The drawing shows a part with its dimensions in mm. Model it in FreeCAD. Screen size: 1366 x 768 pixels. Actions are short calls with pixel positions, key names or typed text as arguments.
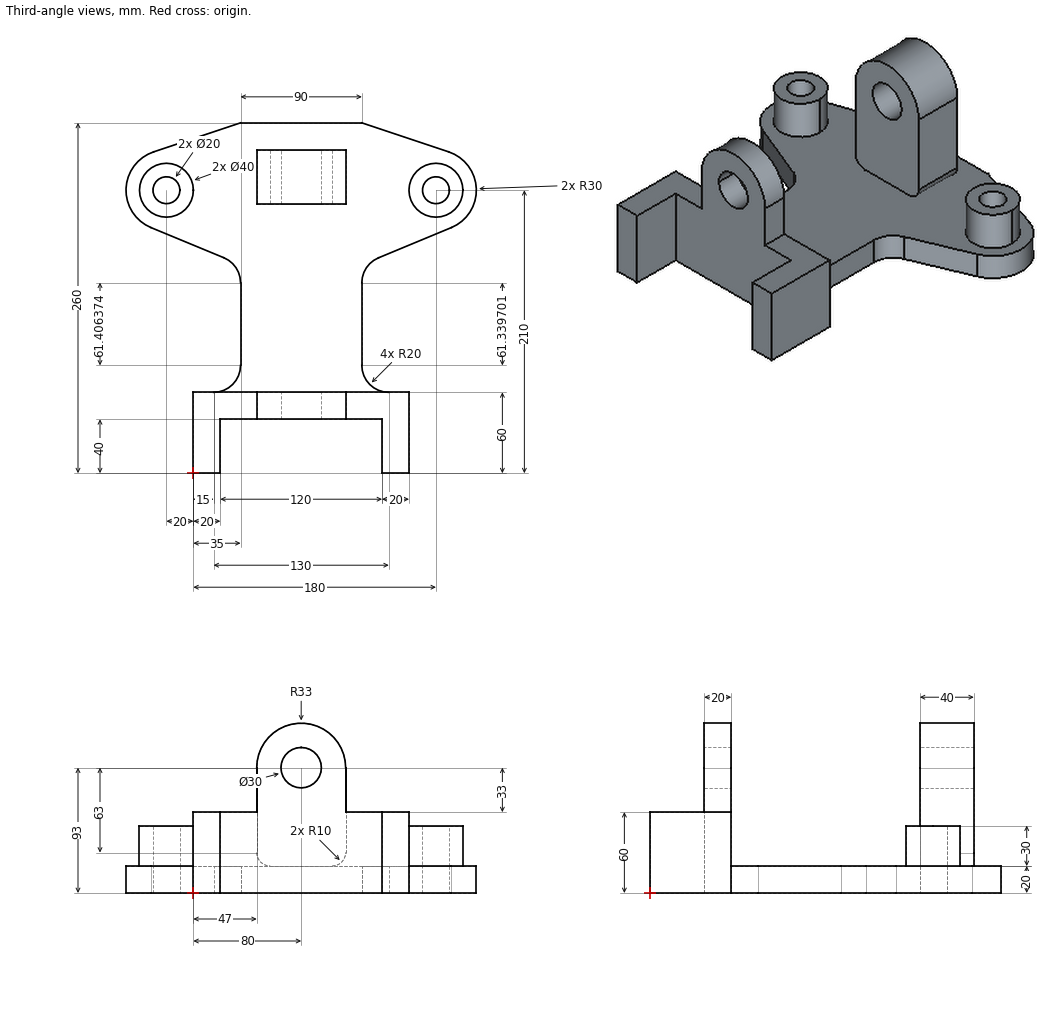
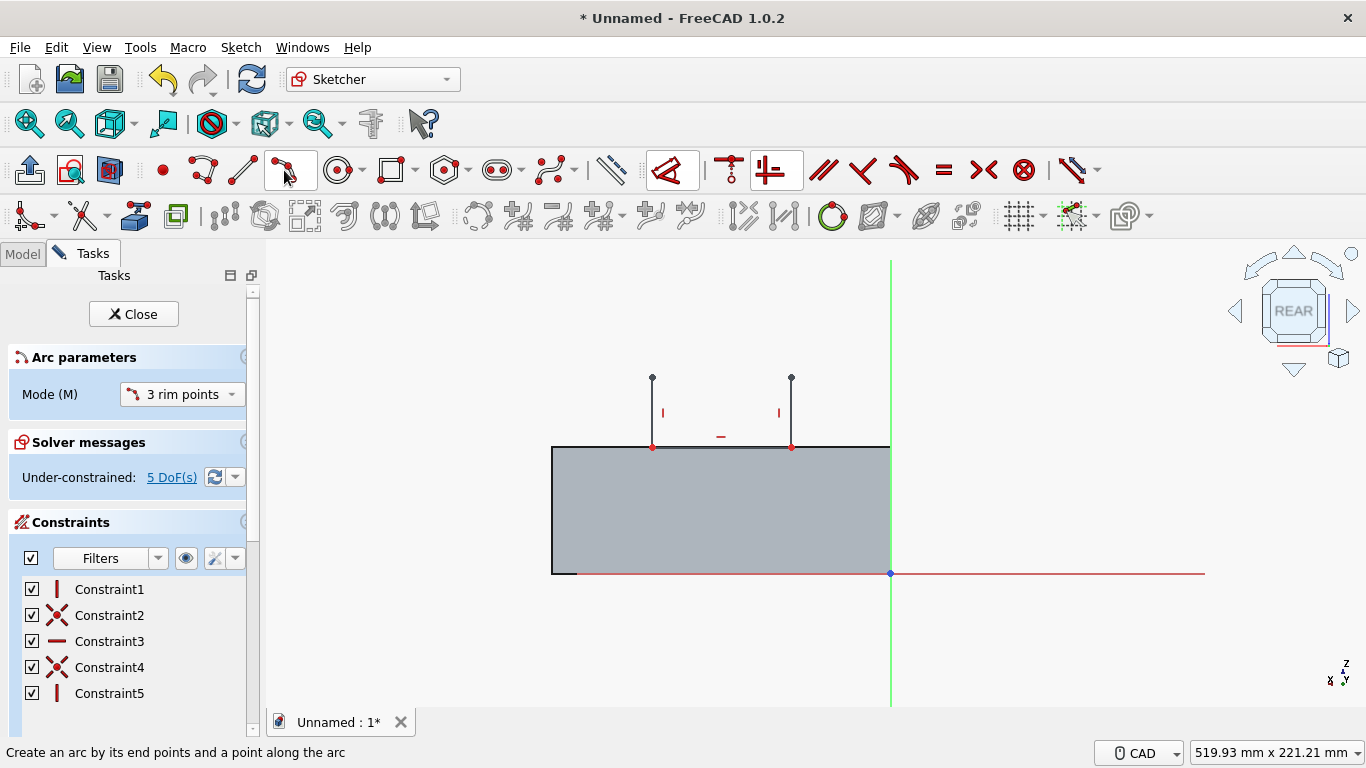
click(791, 378)
click(652, 378)
click(721, 307)
key(Escape)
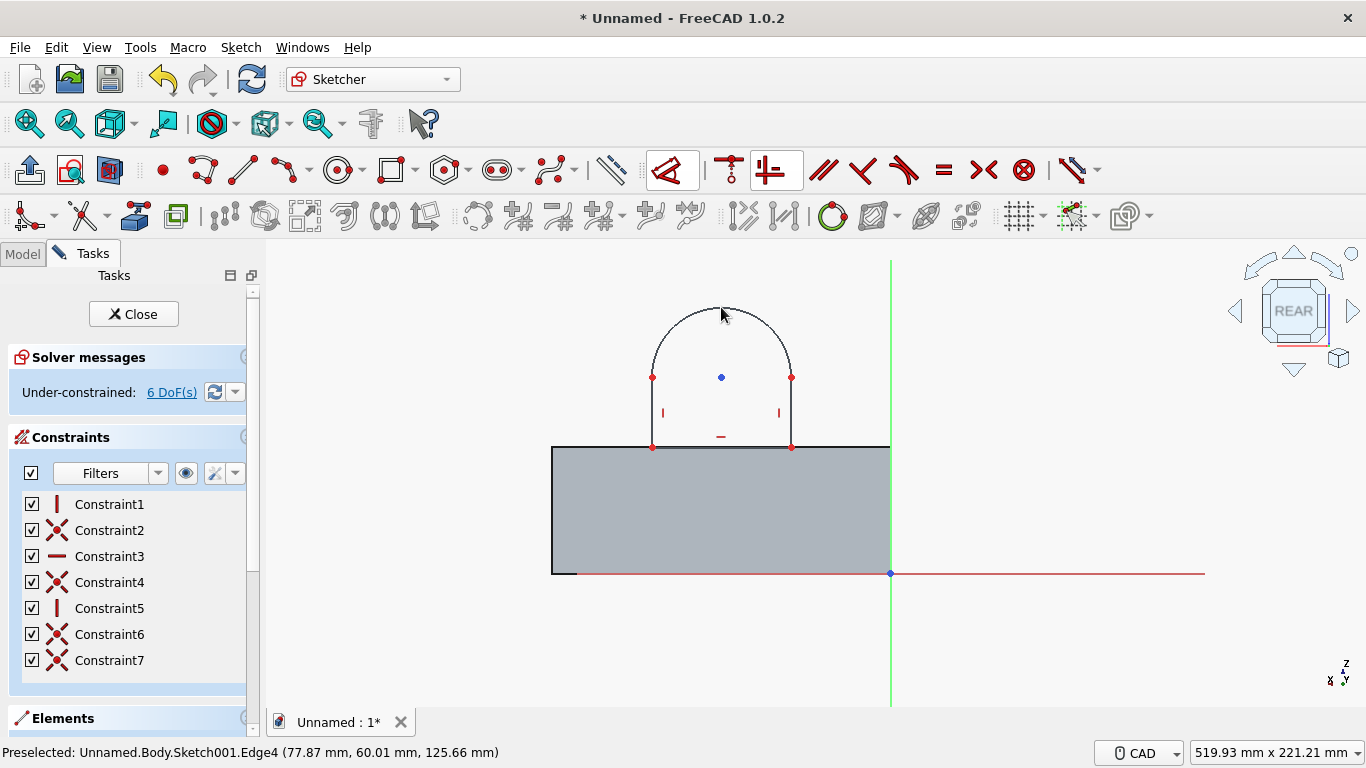
click(652, 399)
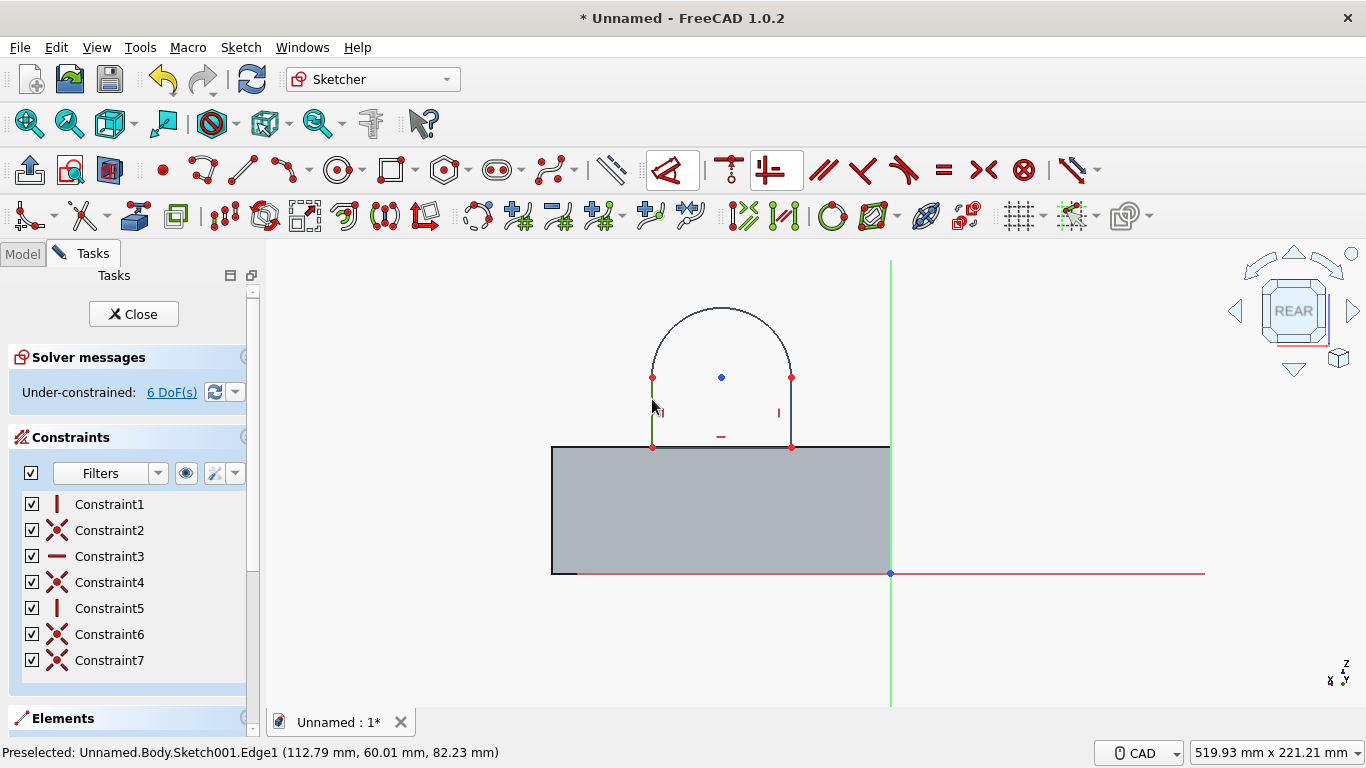
click(763, 321)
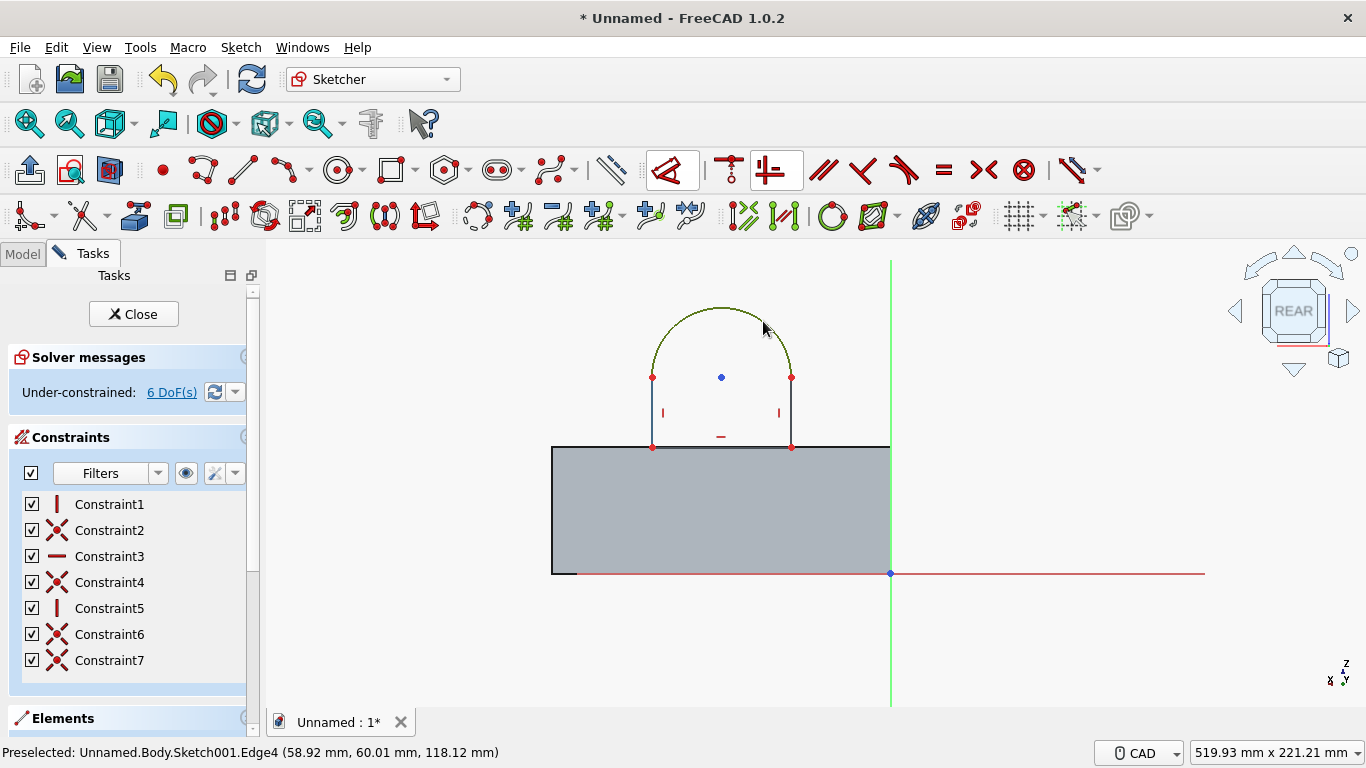
click(904, 170)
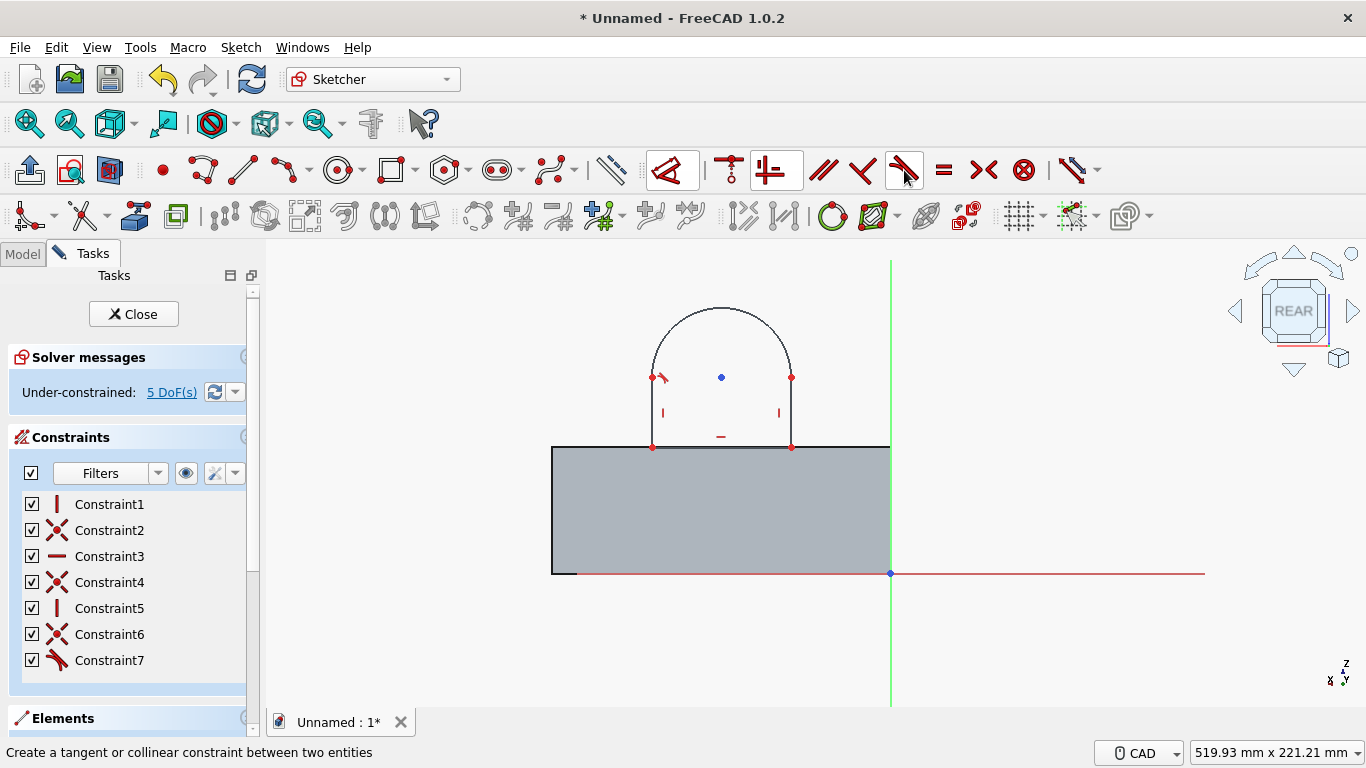
click(791, 427)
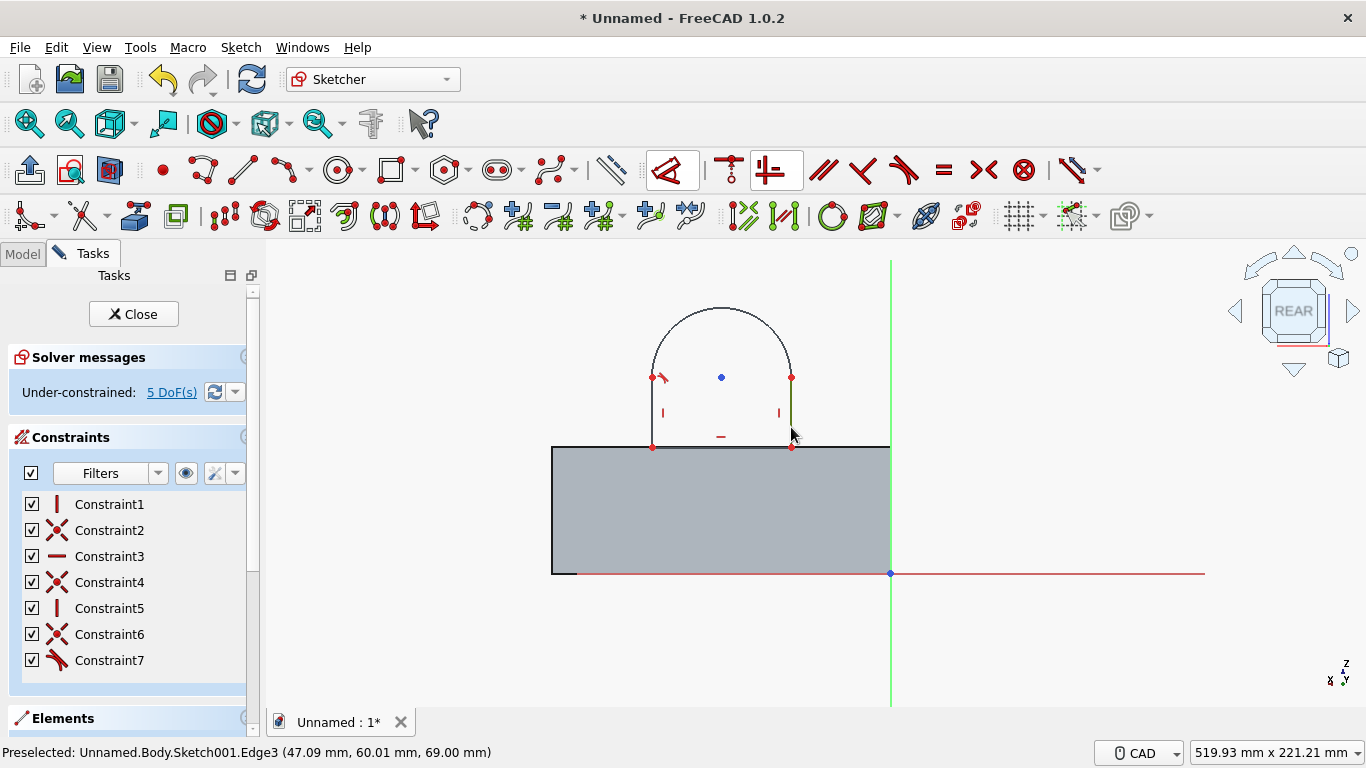
click(763, 321)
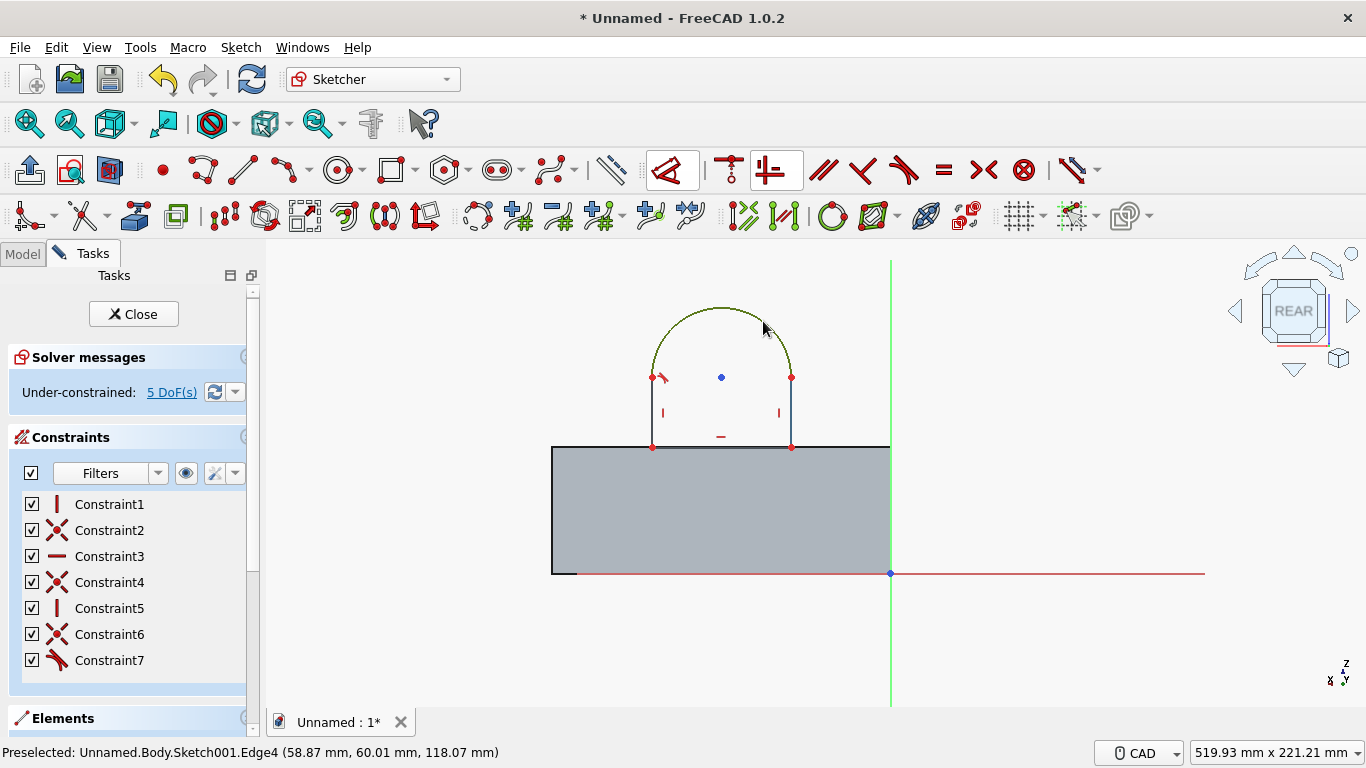
click(904, 170)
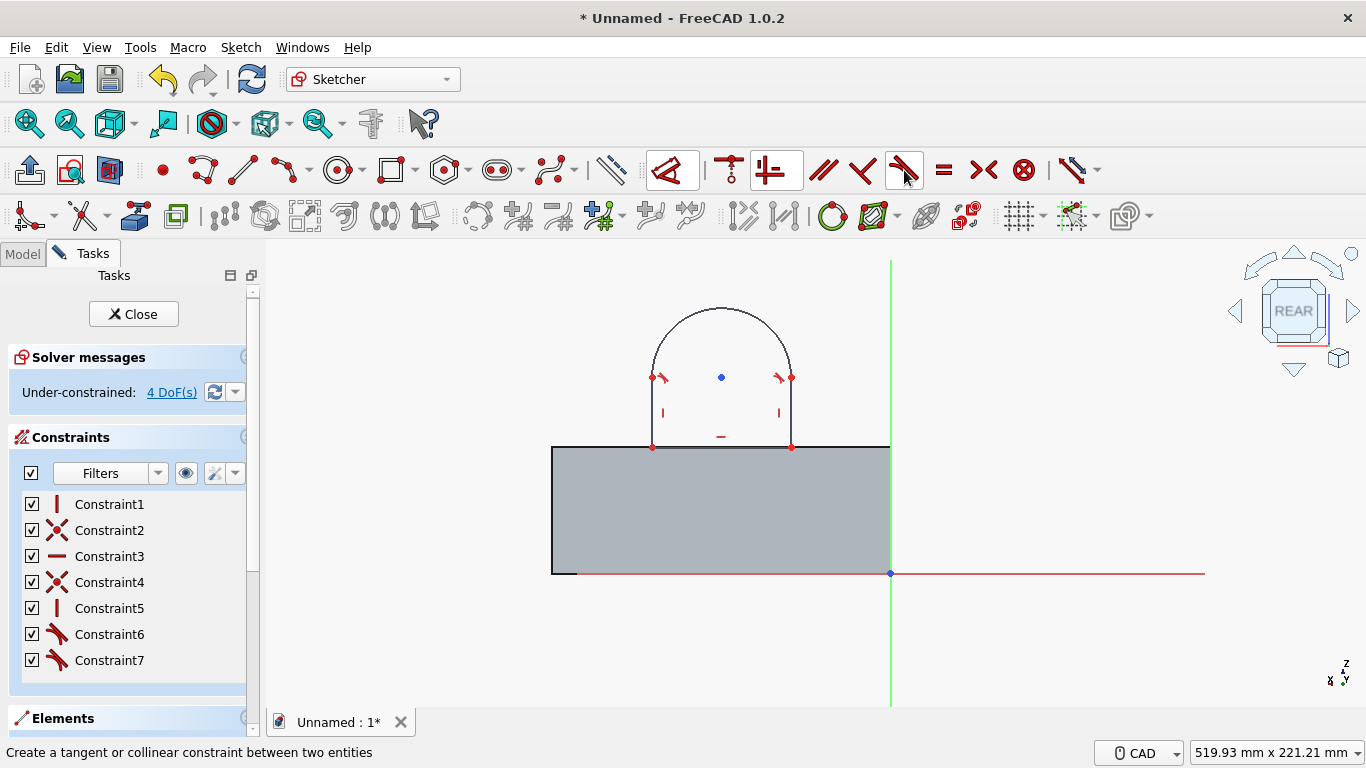
click(762, 322)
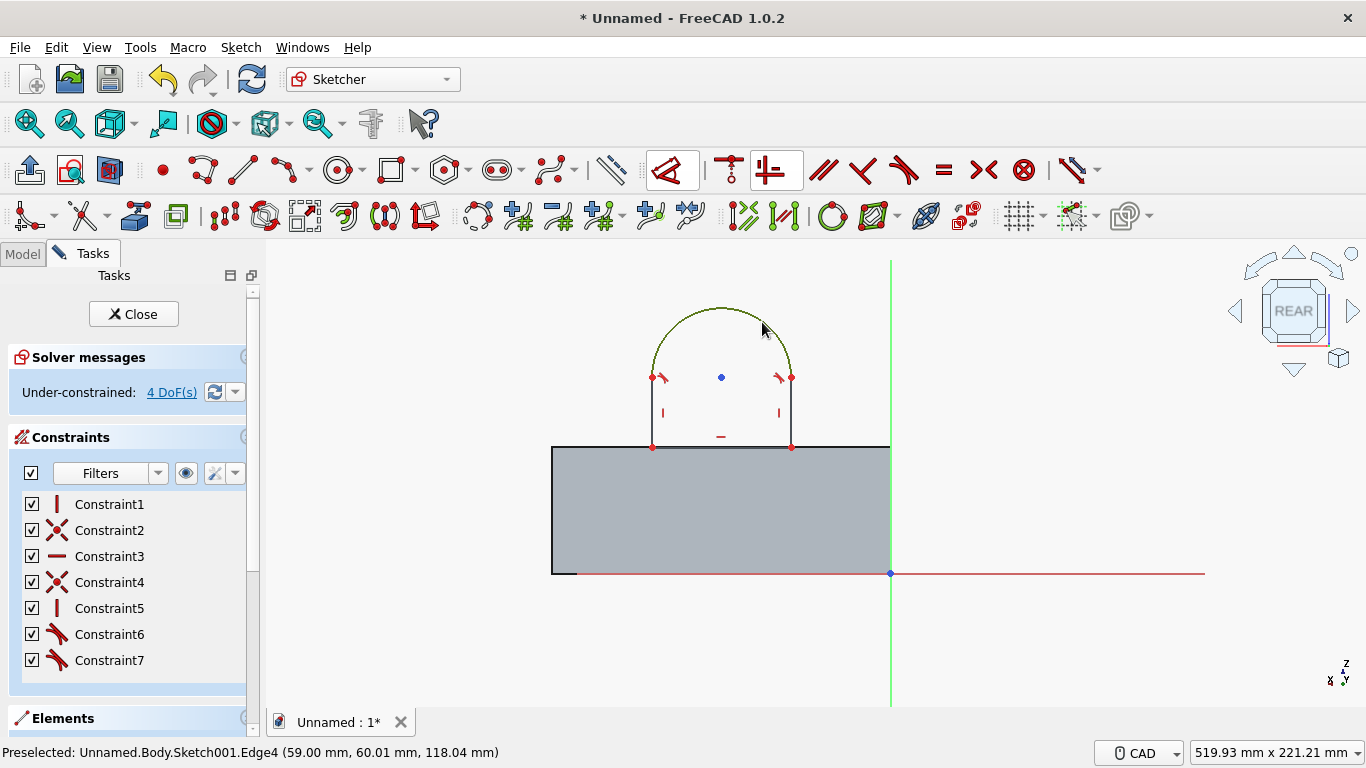
key(k)
key(r)